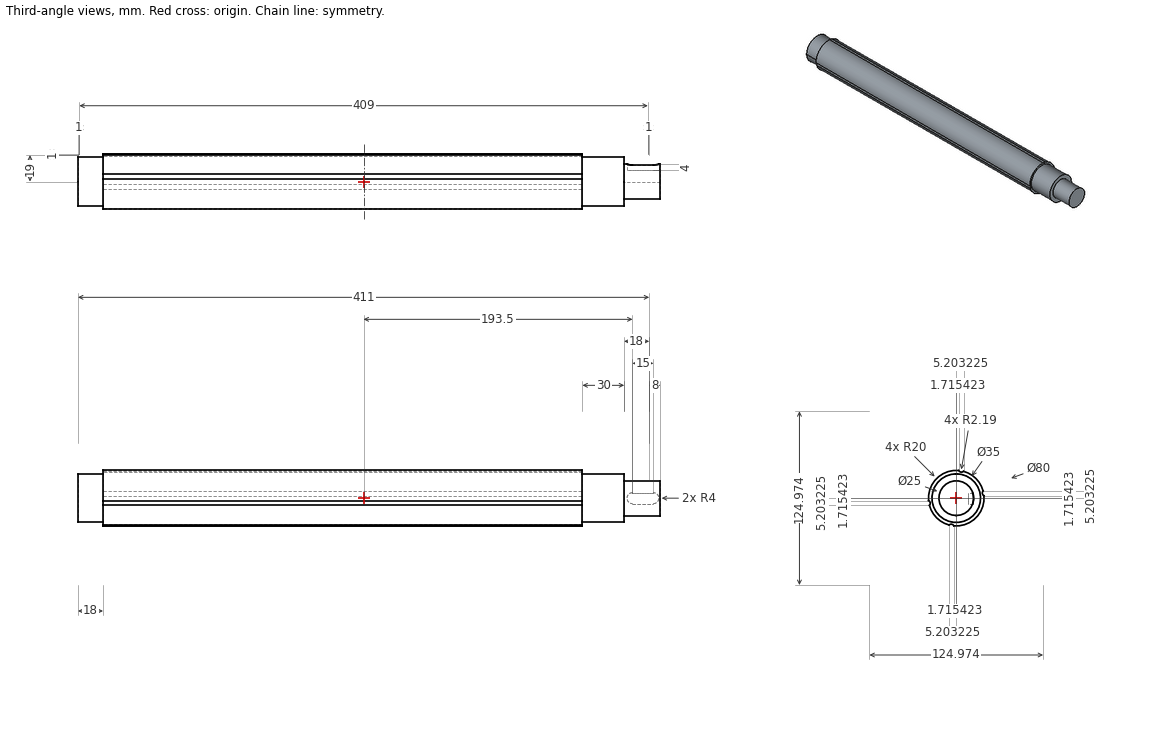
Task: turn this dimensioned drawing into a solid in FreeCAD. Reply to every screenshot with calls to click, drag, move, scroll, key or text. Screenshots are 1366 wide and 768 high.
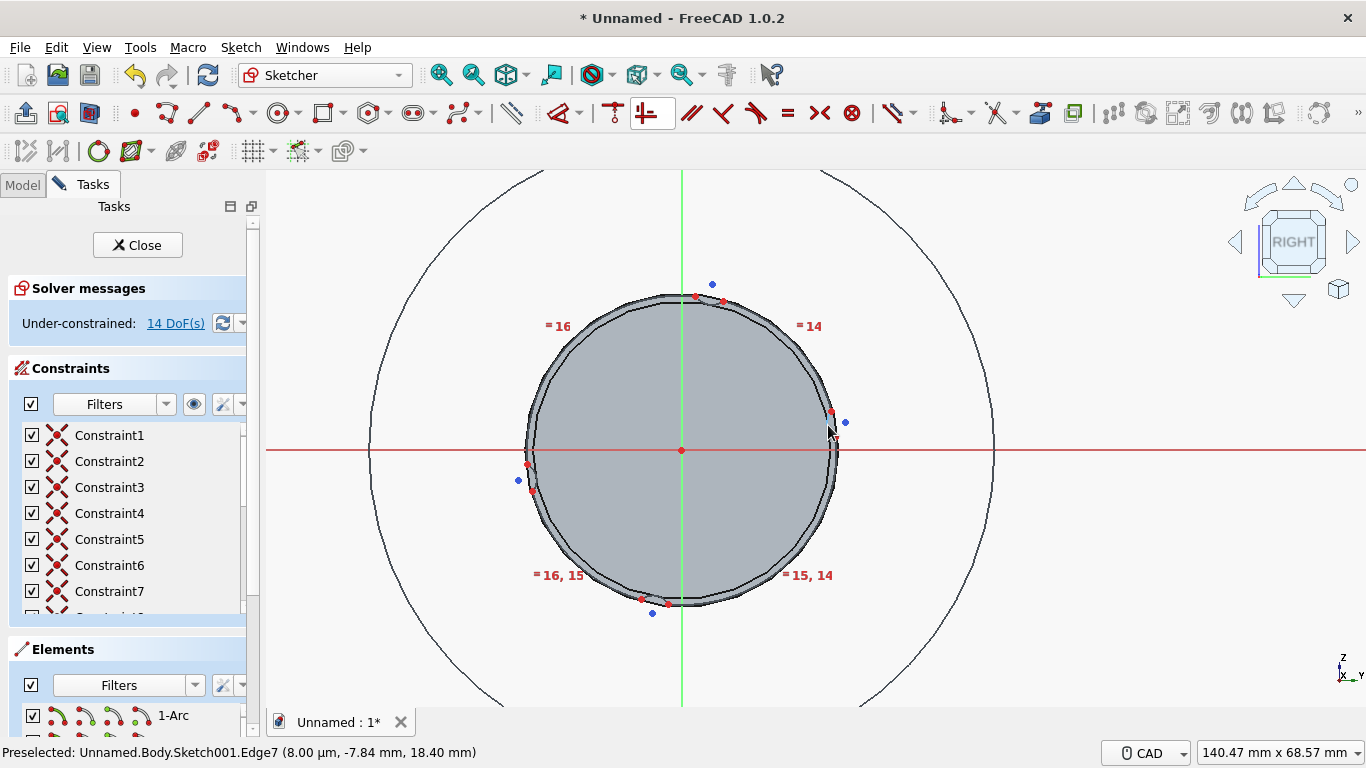
click(828, 425)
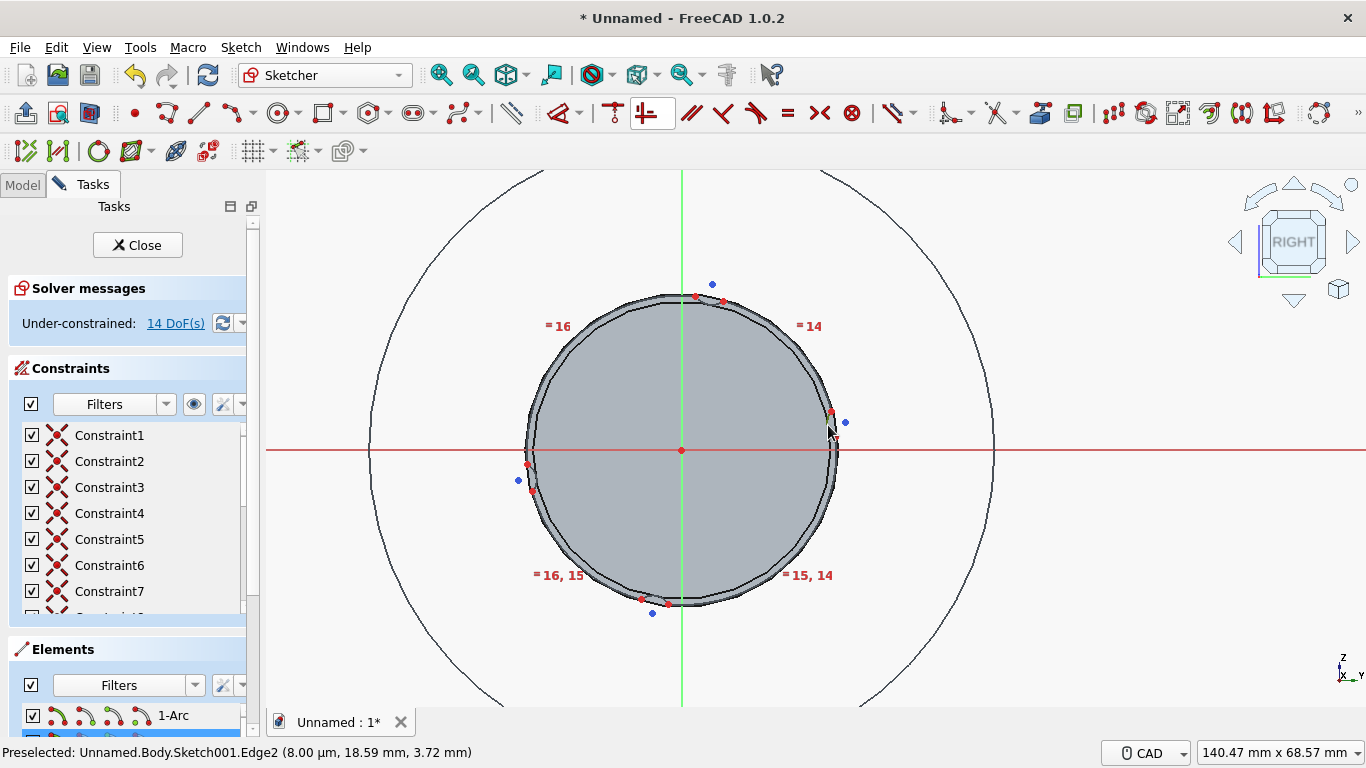
scroll(662, 598, up, 2)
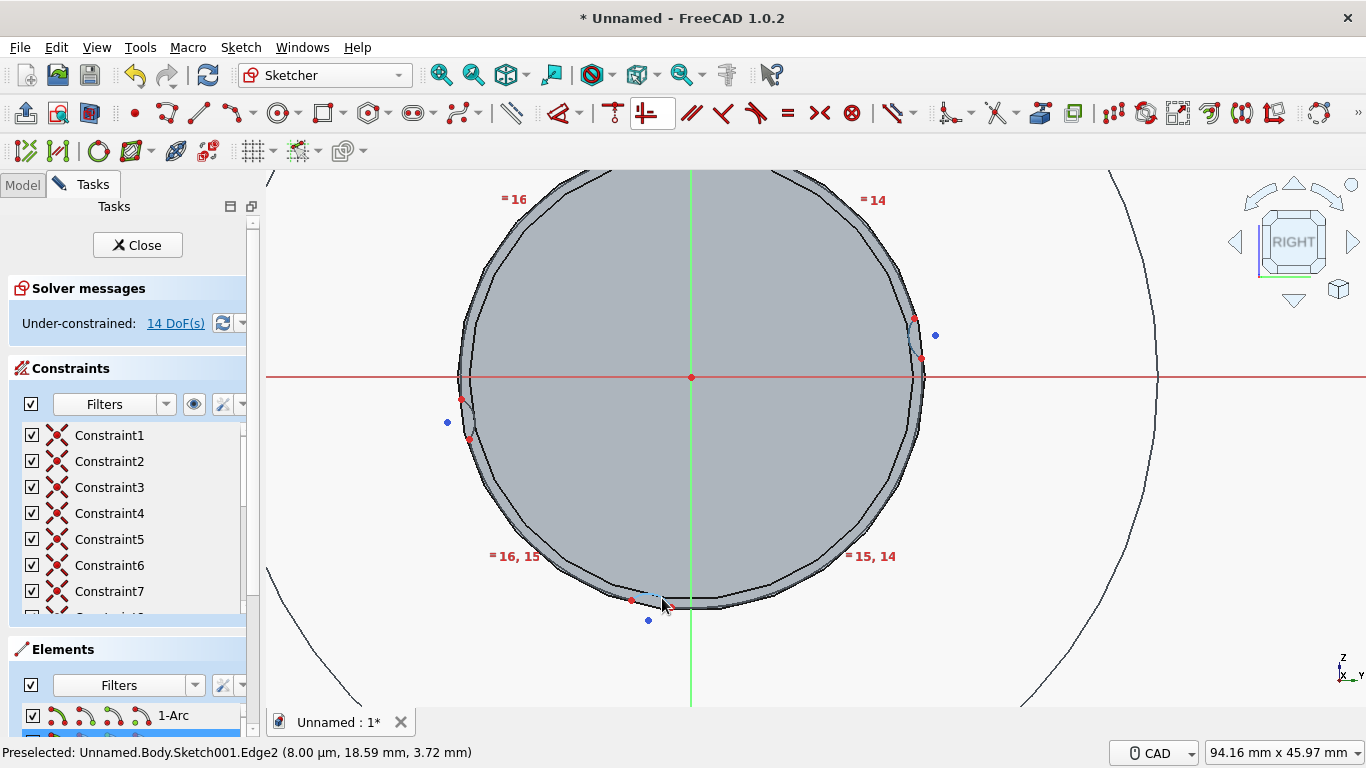
click(662, 597)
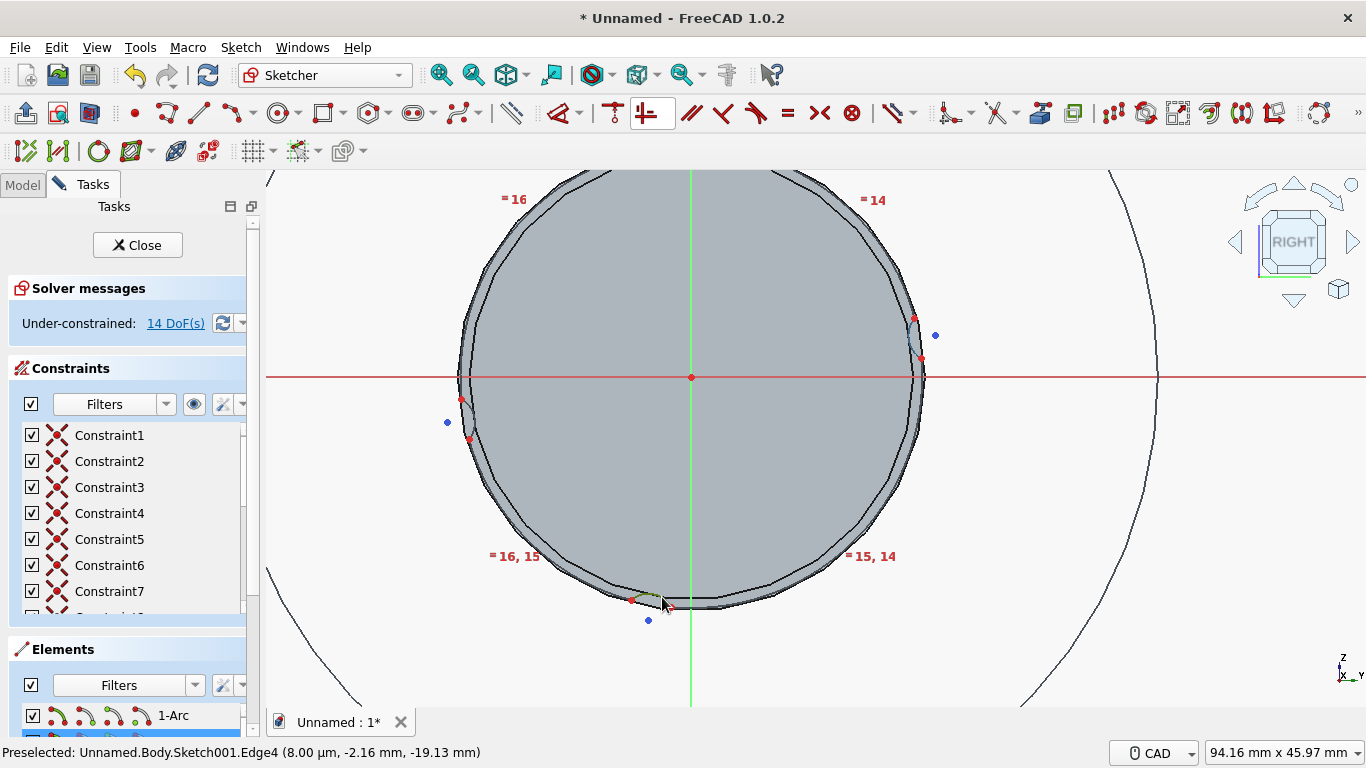
click(475, 427)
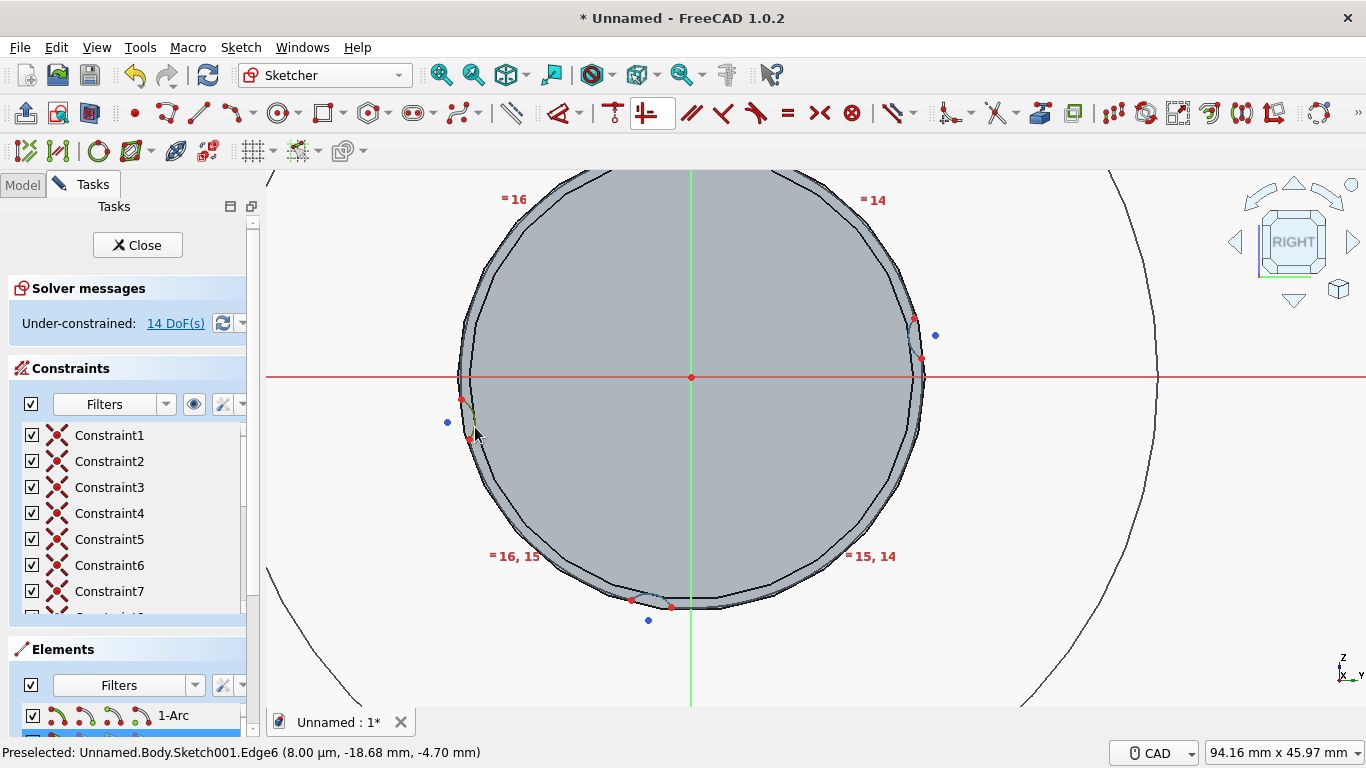
scroll(780, 474, down, 5)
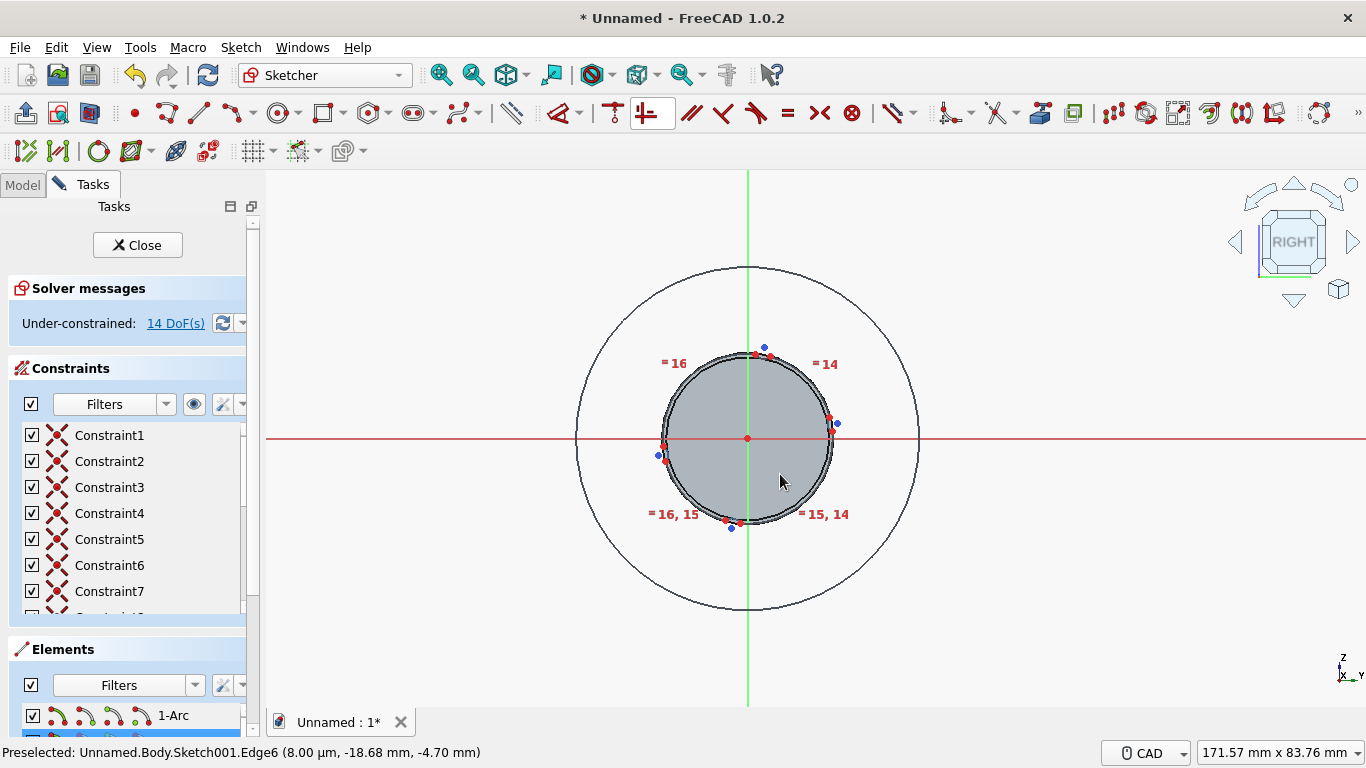
scroll(759, 358, up, 5)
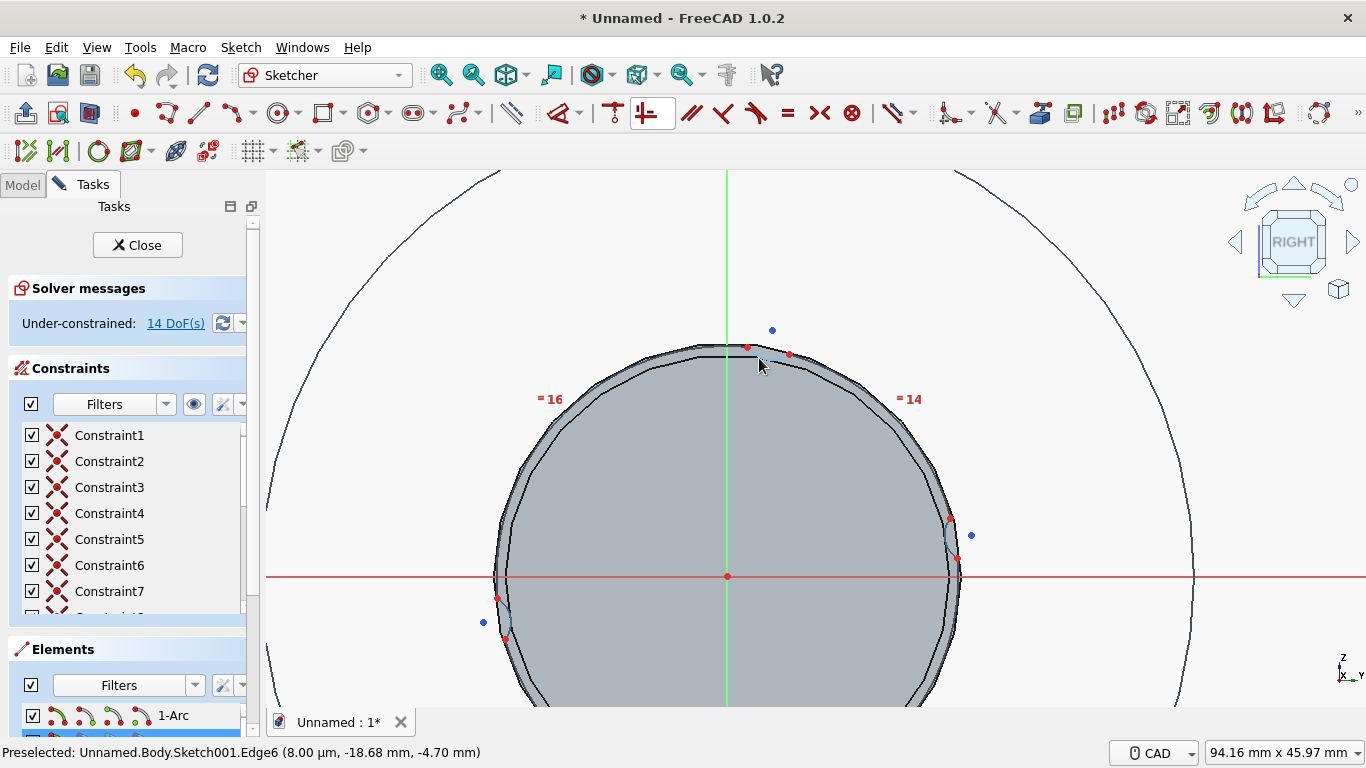
click(758, 356)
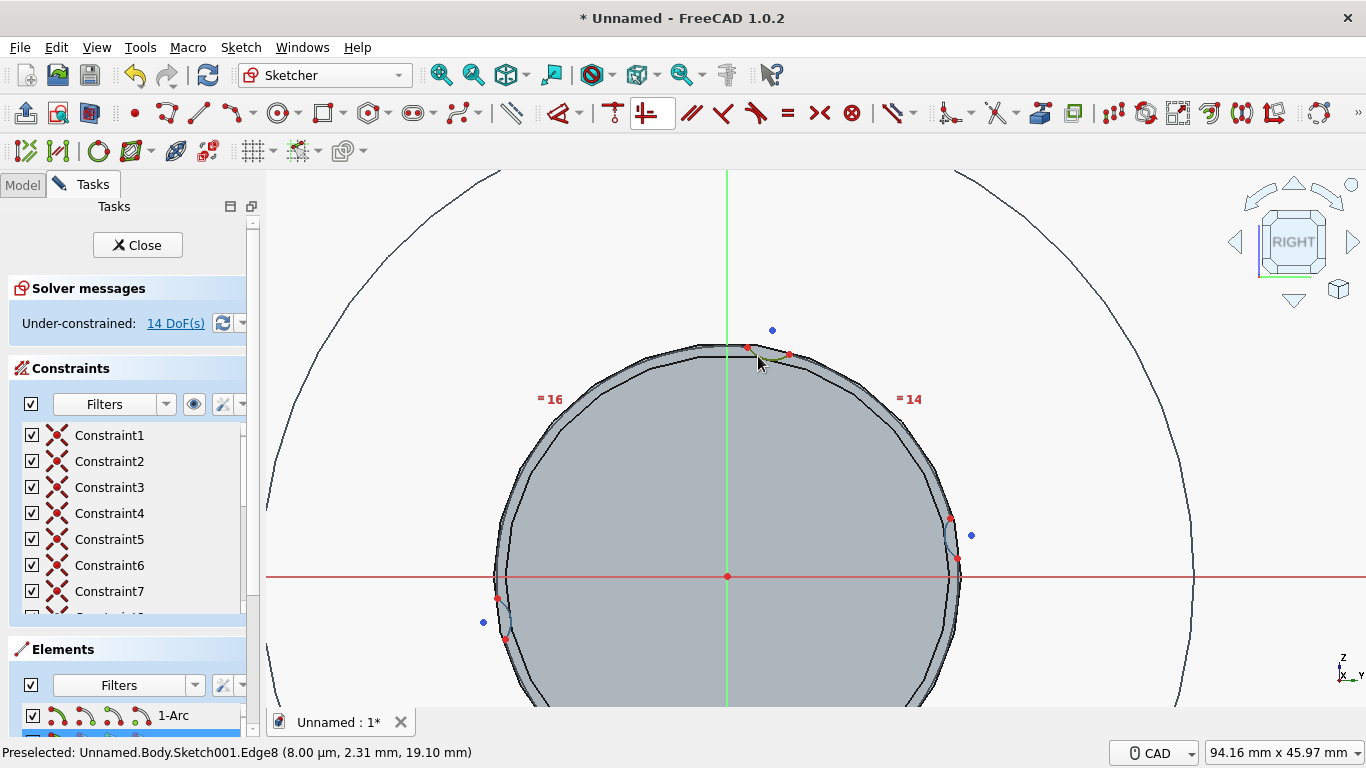
key(e)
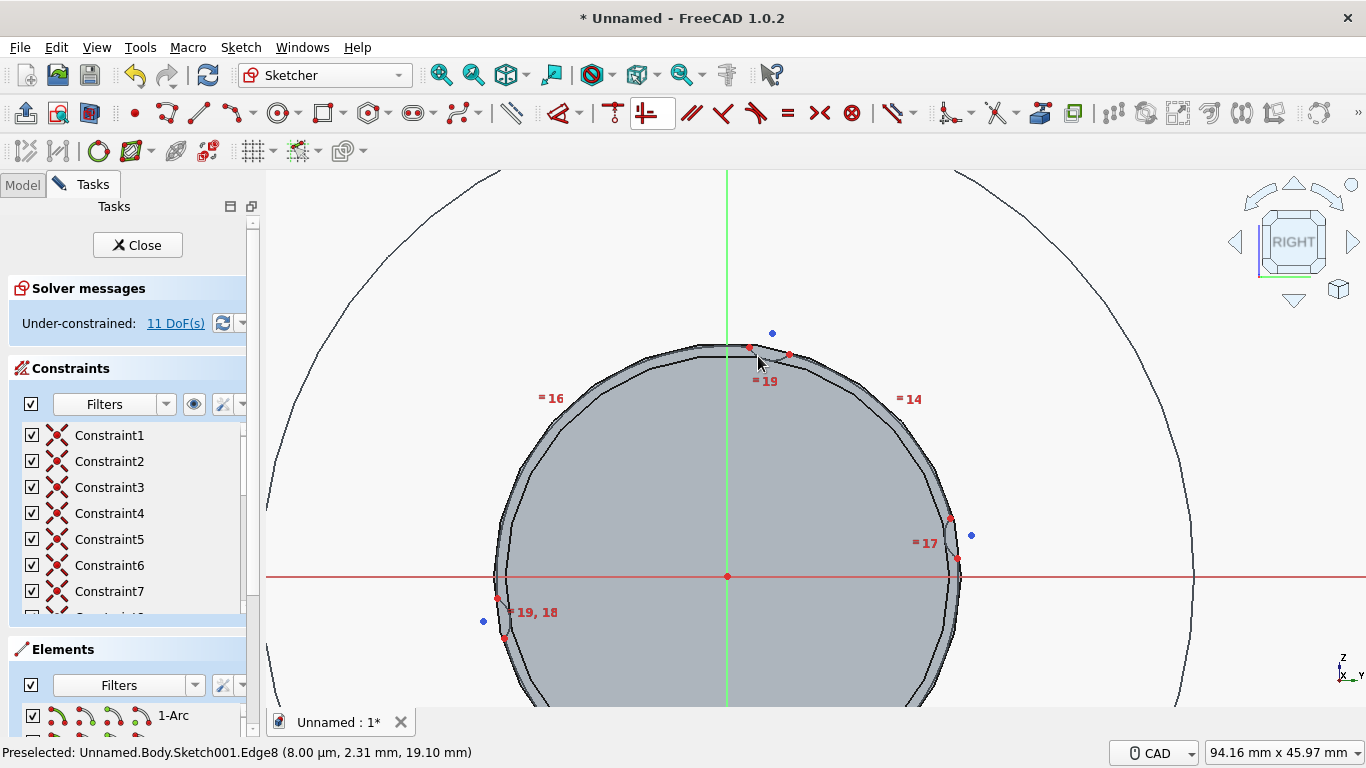
key(d)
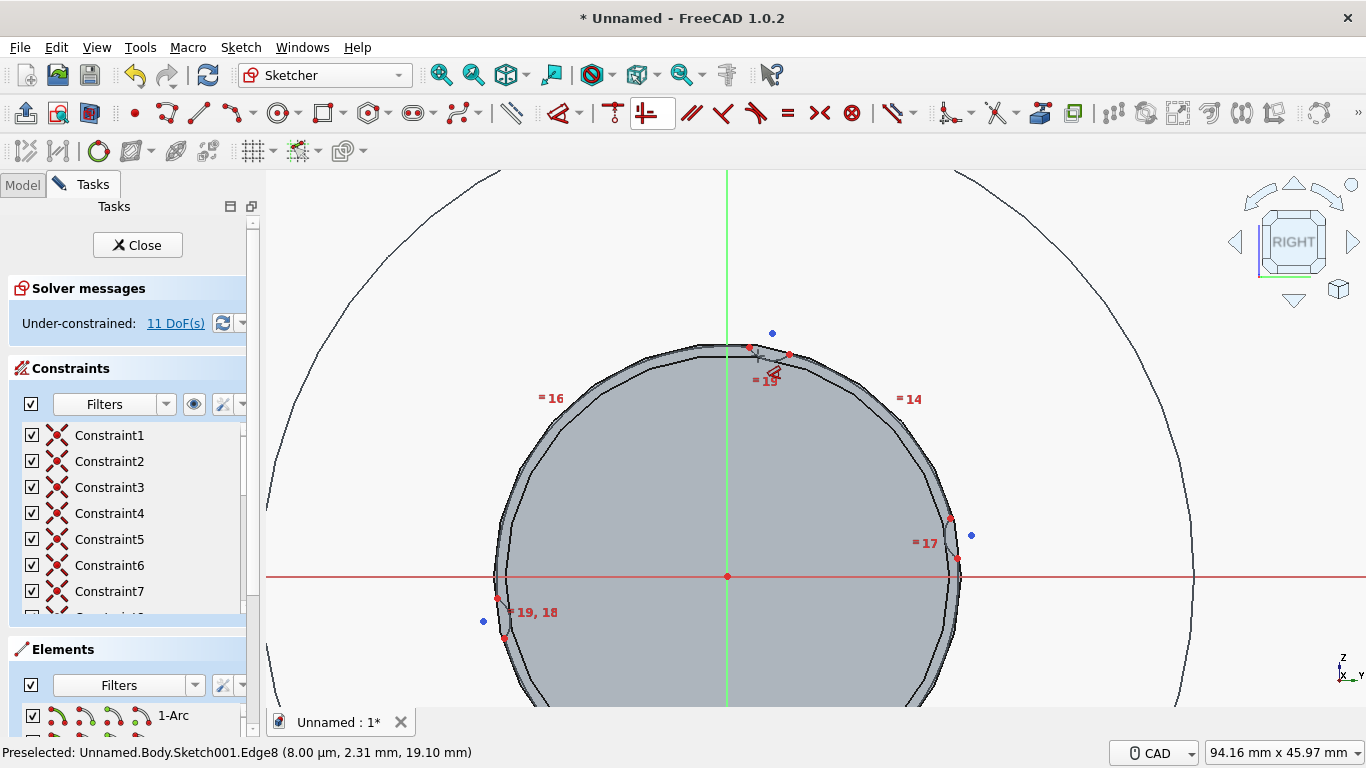
click(922, 453)
click(949, 436)